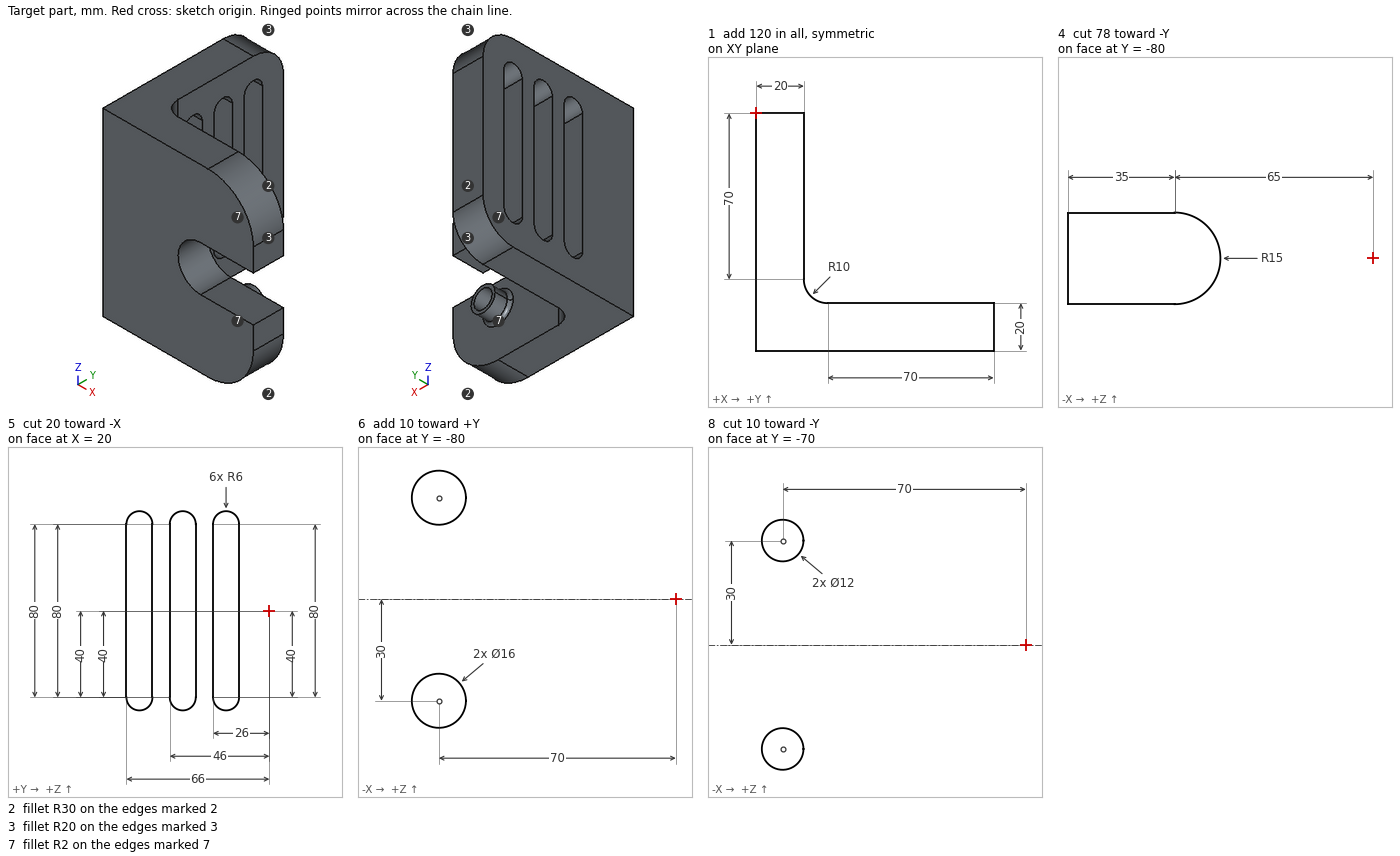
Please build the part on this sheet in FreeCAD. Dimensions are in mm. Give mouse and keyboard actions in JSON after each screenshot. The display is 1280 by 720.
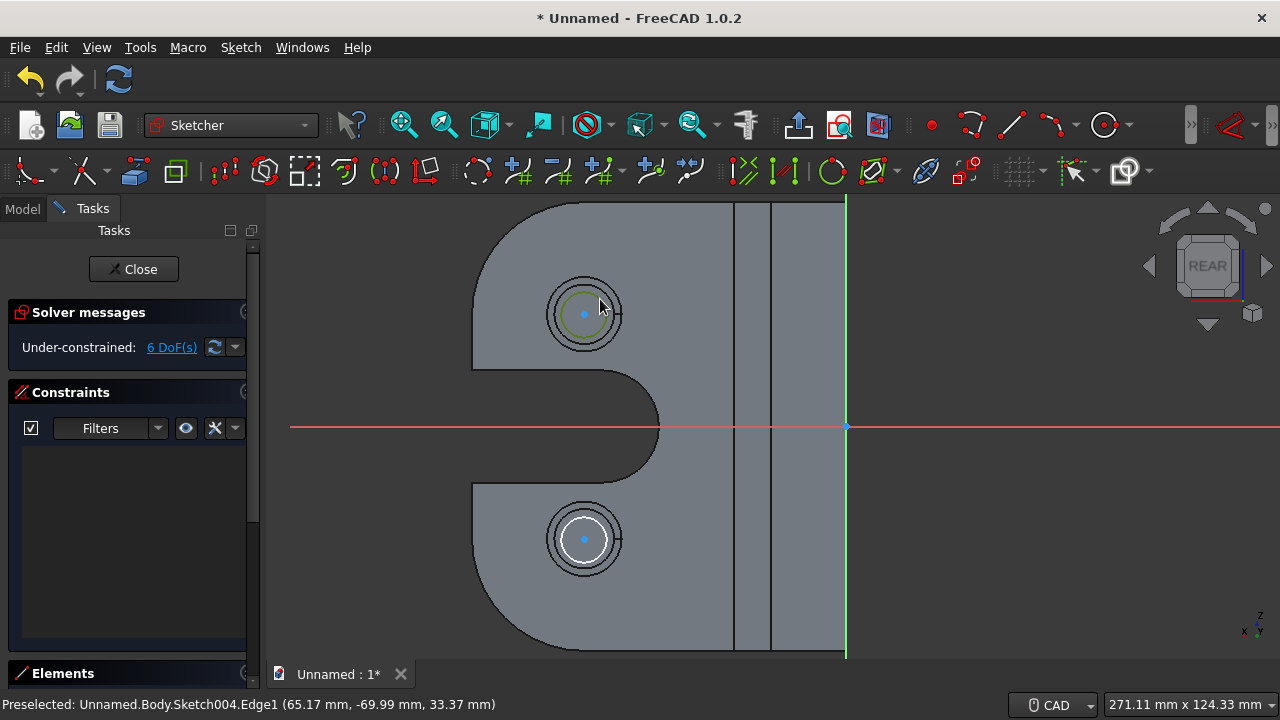
{"action": "left_click", "coordinate": [600, 524]}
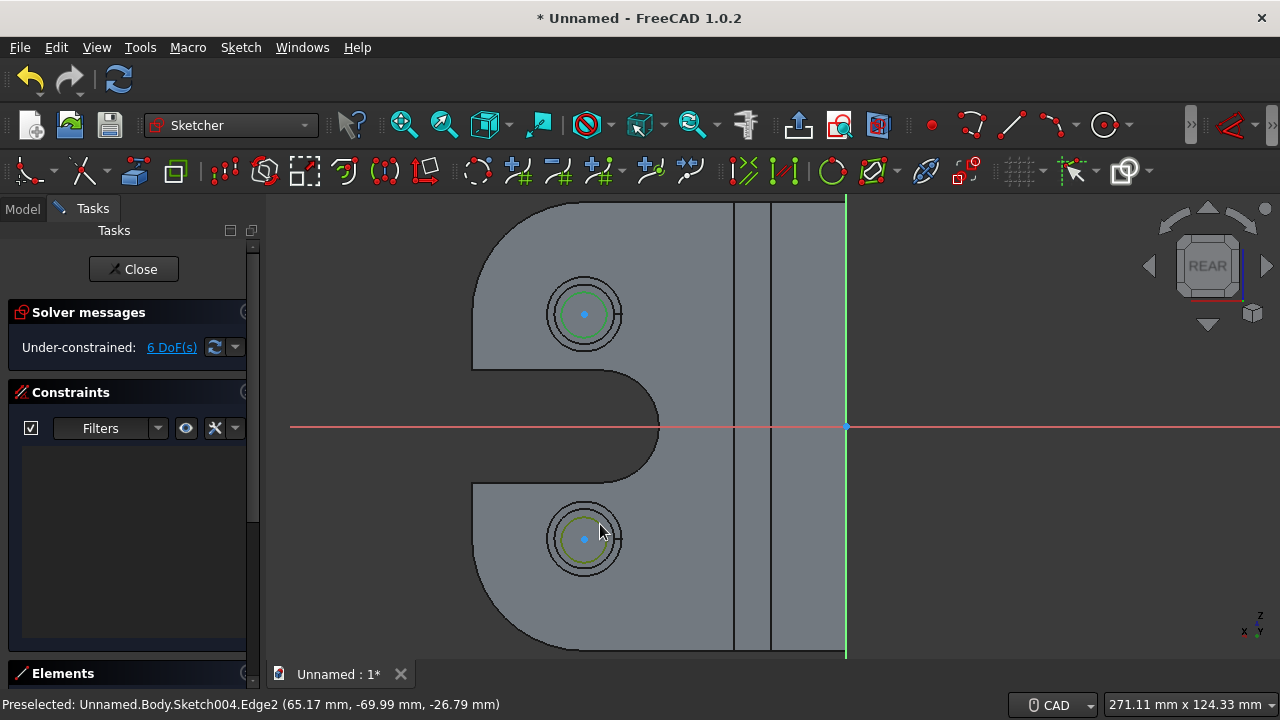
{"action": "key", "text": "e"}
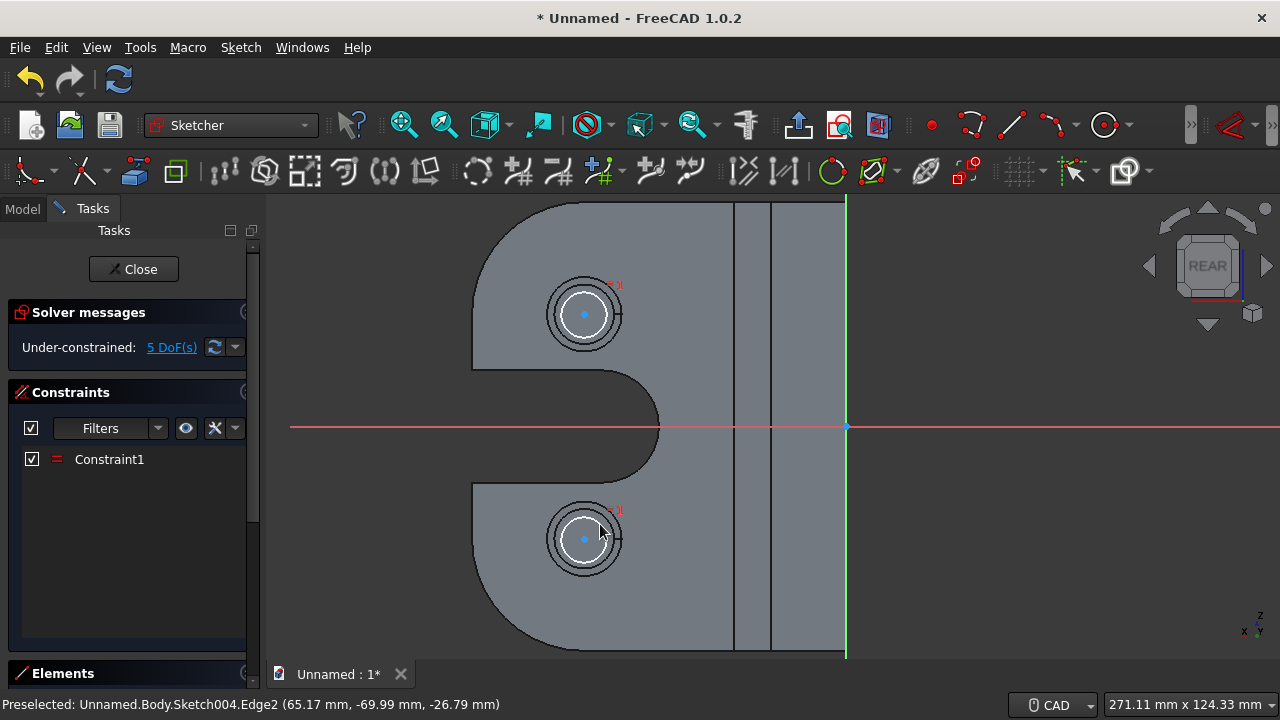
{"action": "left_click", "coordinate": [584, 315]}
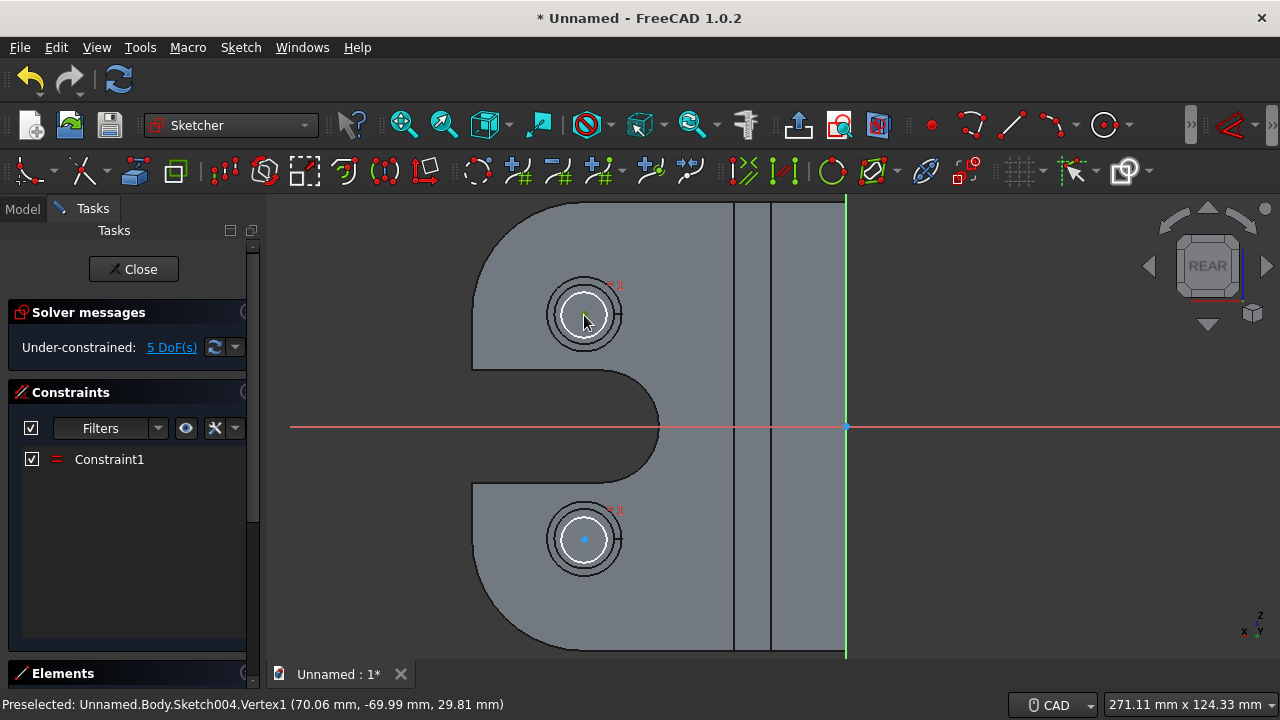
{"action": "left_click", "coordinate": [584, 540]}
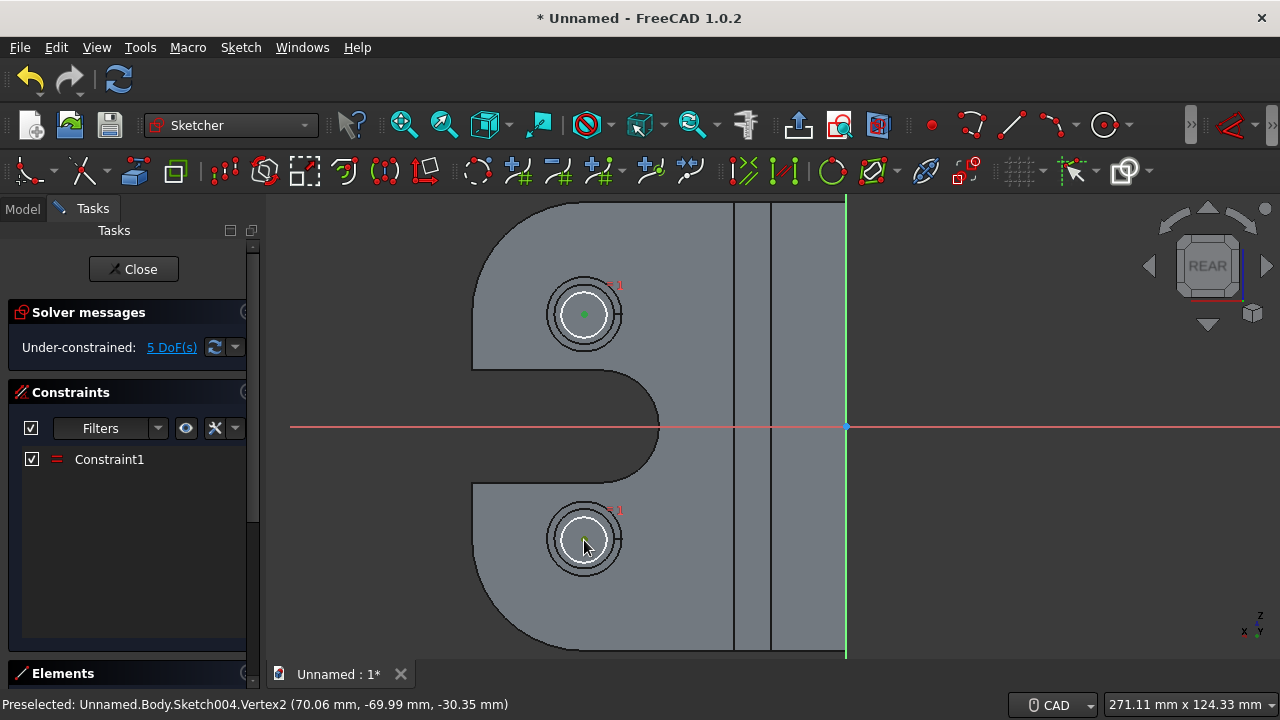
{"action": "left_click", "coordinate": [353, 426]}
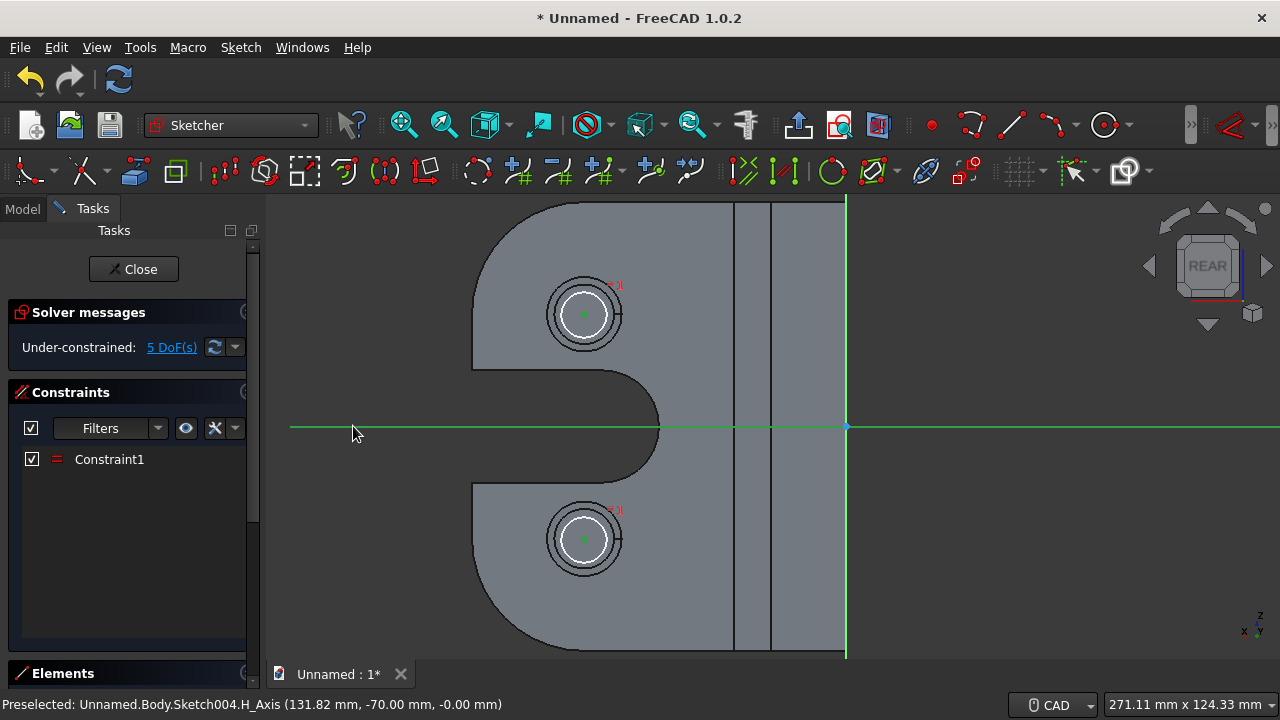
{"action": "key", "text": "s"}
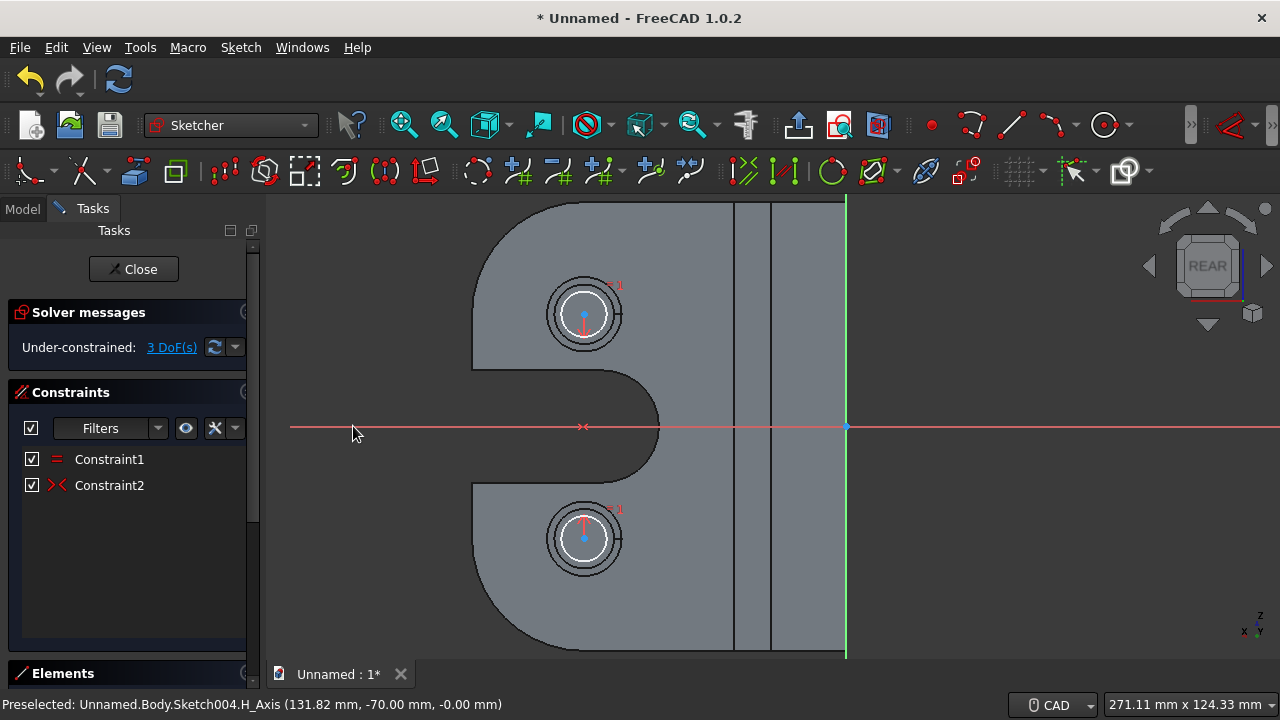
{"action": "left_click", "coordinate": [1230, 126]}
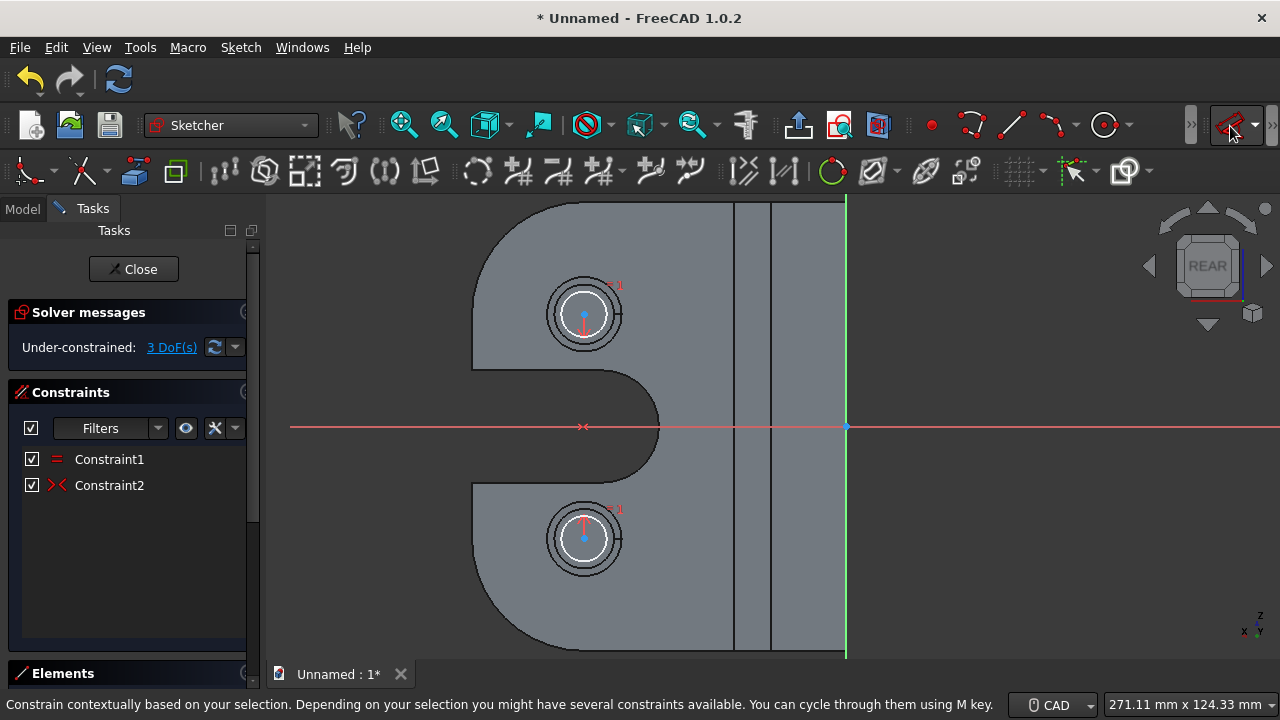
{"action": "left_click", "coordinate": [600, 298]}
{"action": "left_click", "coordinate": [622, 275]}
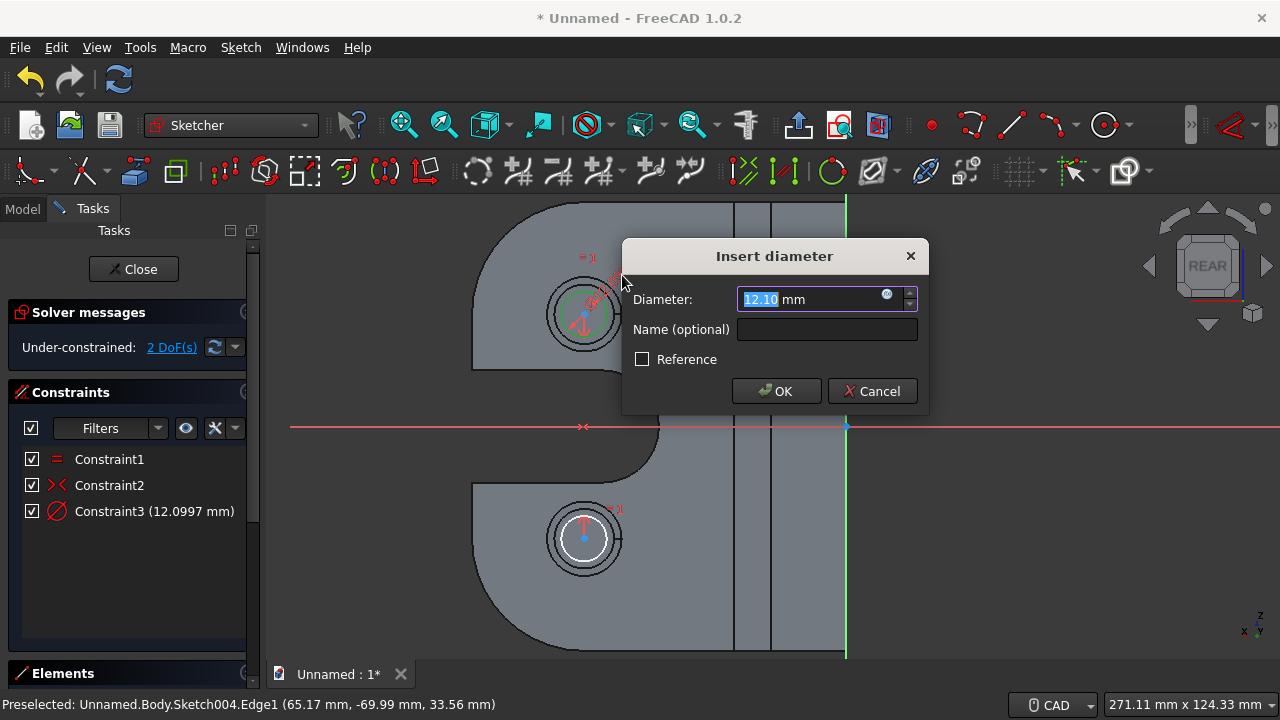
{"action": "type", "text": "12"}
{"action": "key", "text": "Return"}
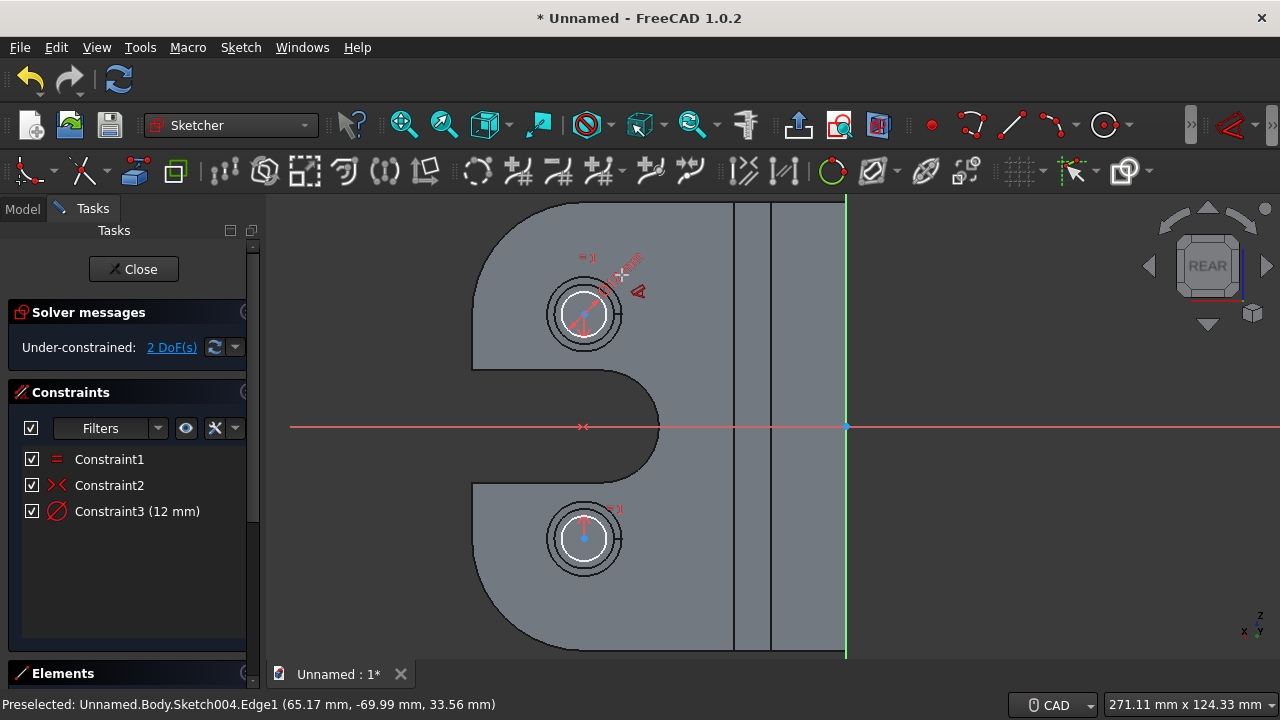
{"action": "left_click", "coordinate": [584, 314]}
{"action": "left_click", "coordinate": [715, 280]}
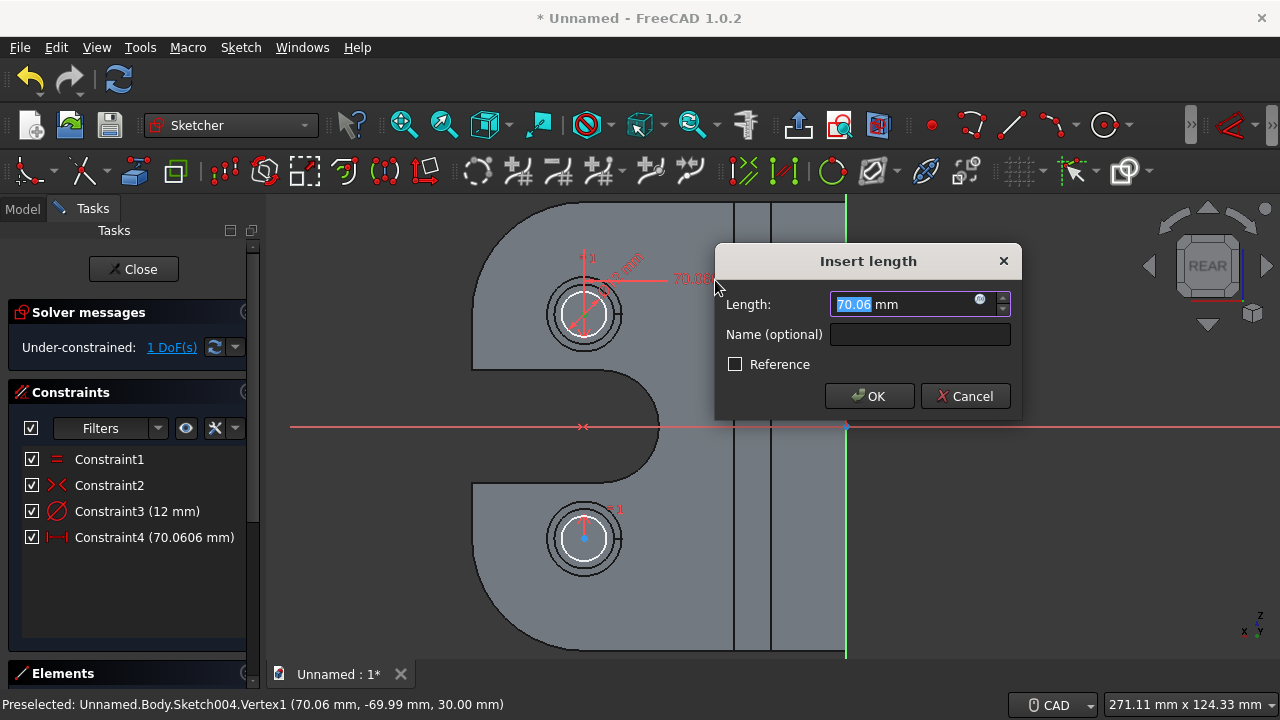
{"action": "type", "text": "70"}
{"action": "key", "text": "Return"}